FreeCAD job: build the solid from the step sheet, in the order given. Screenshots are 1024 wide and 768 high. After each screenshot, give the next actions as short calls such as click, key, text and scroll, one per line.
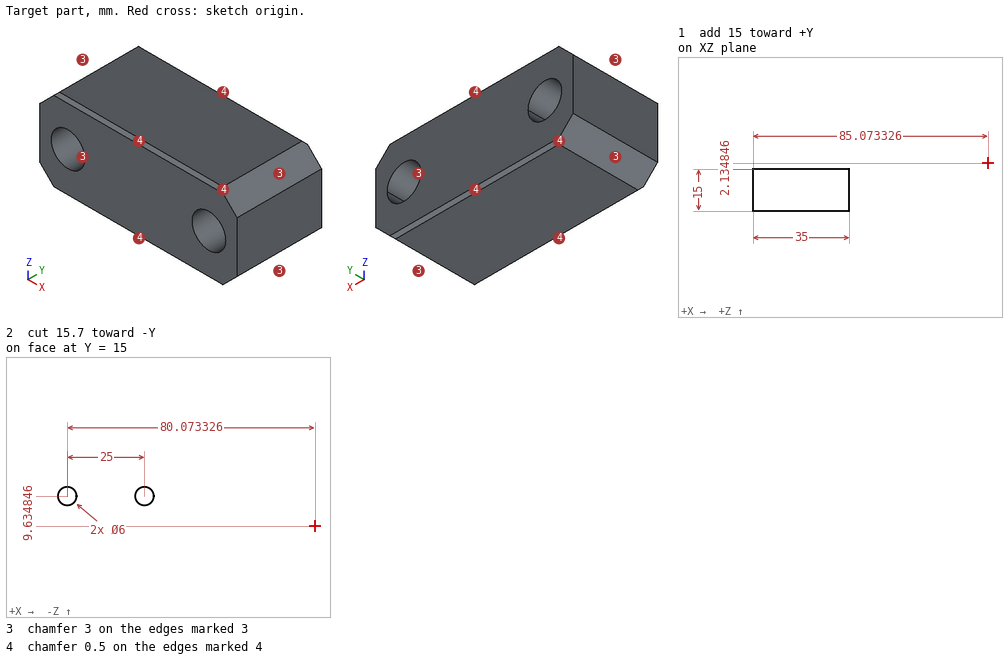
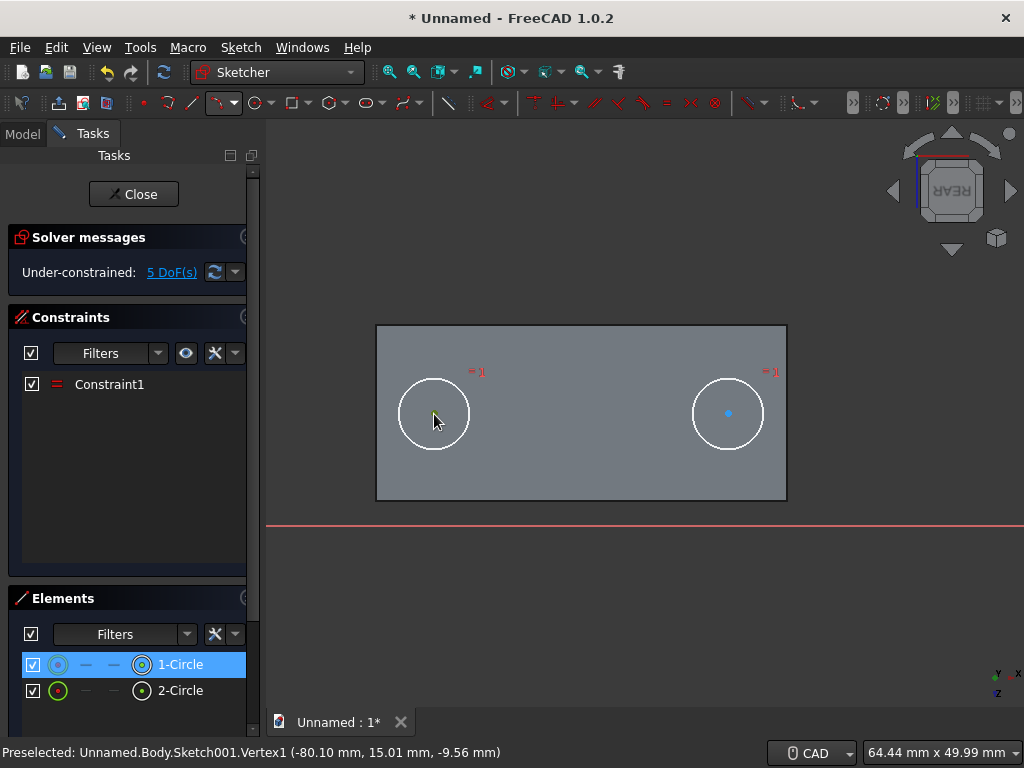
click(728, 414)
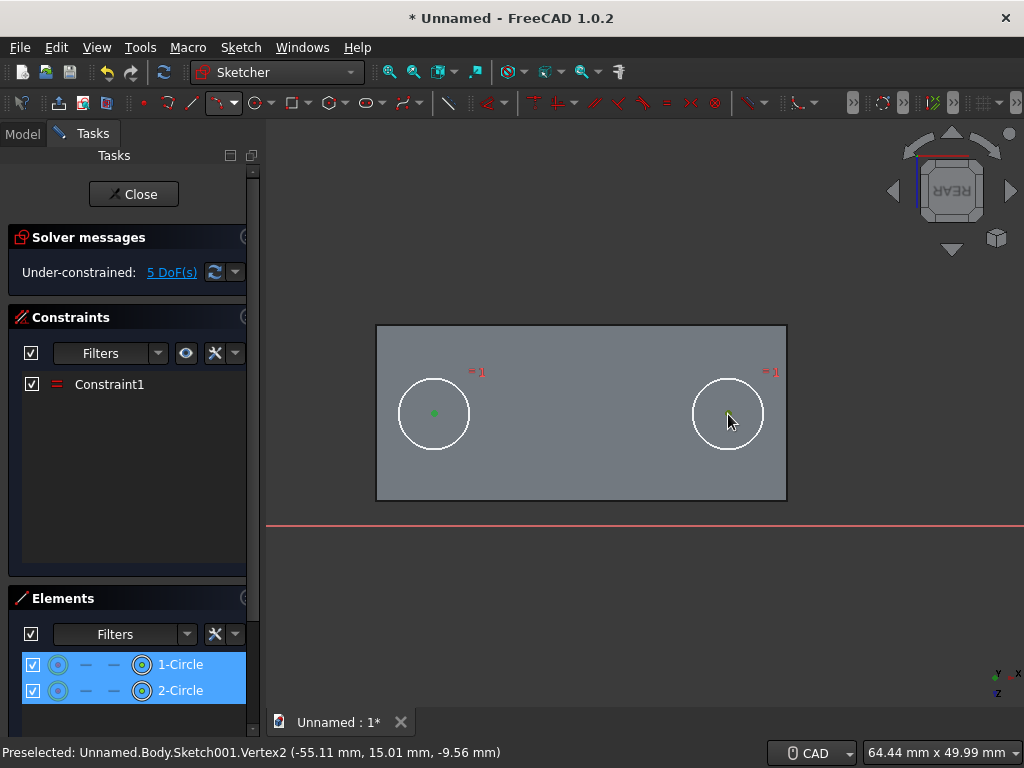
key(h)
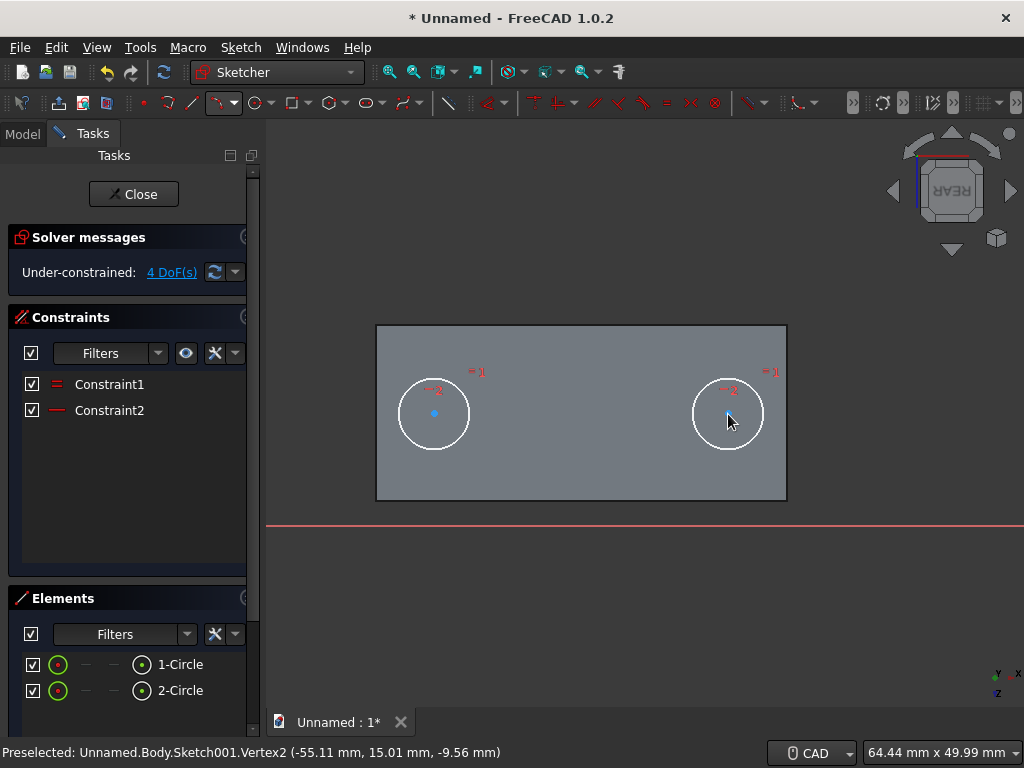
click(459, 389)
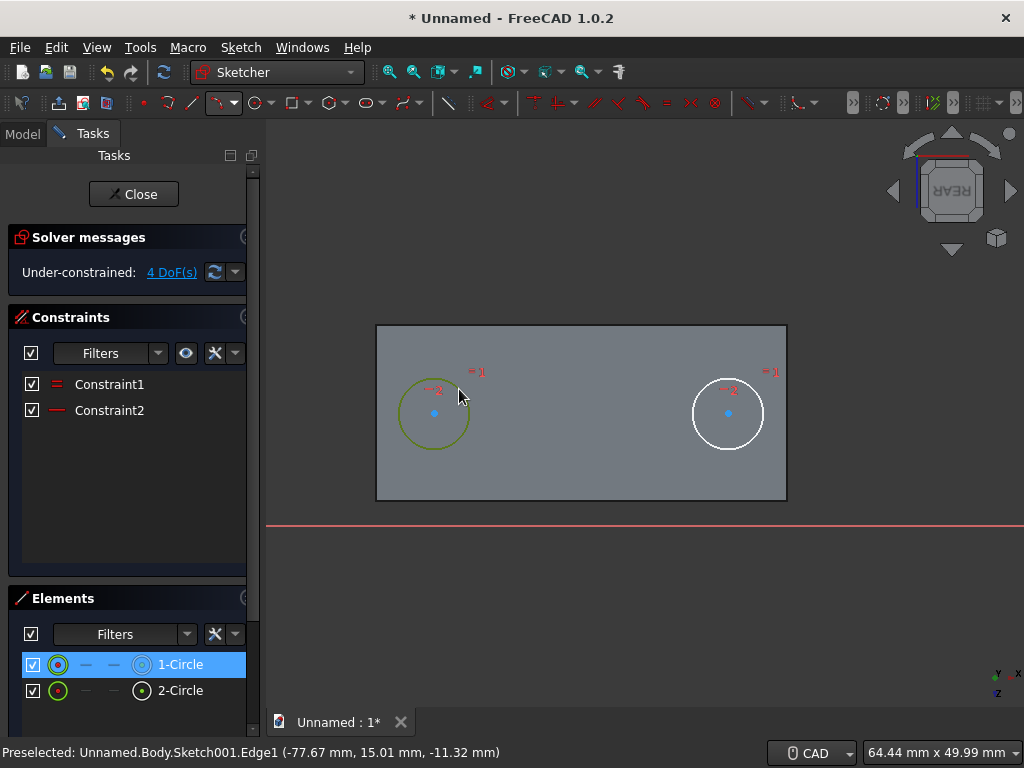
click(506, 104)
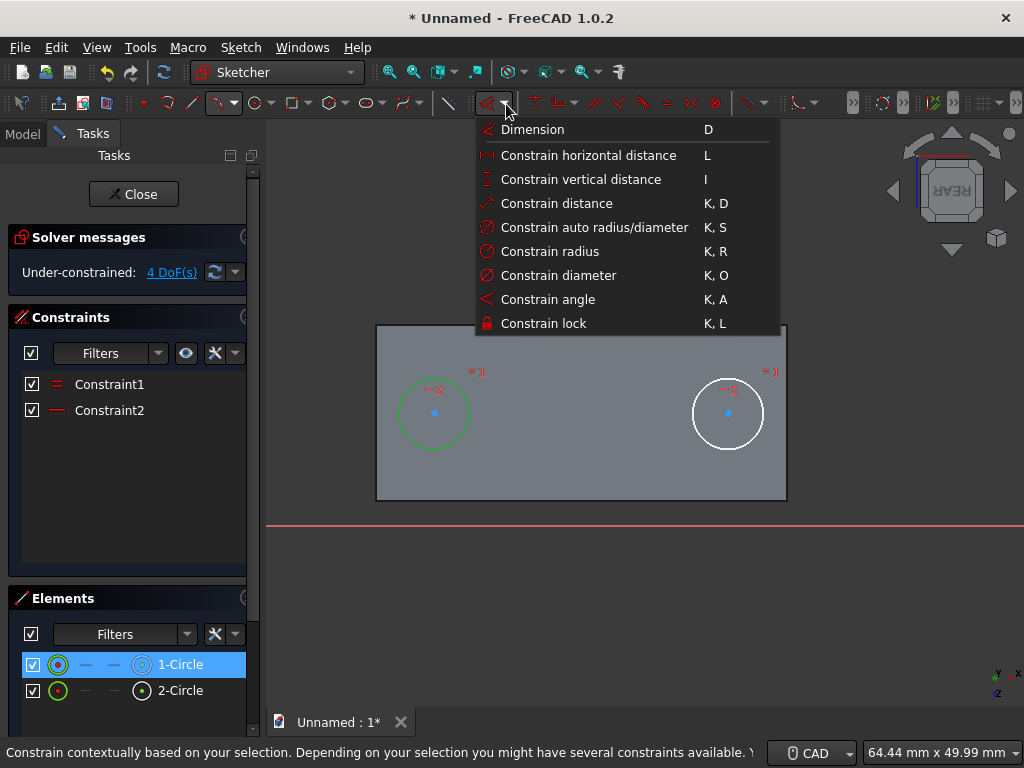
click(628, 275)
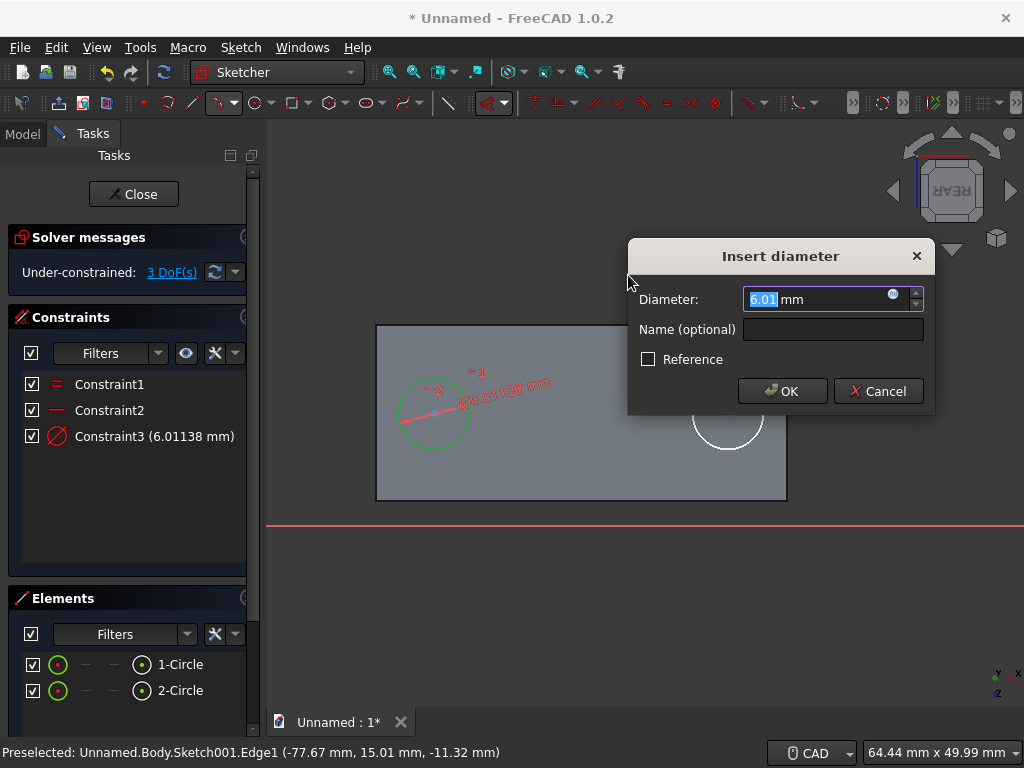
text(6)
key(Return)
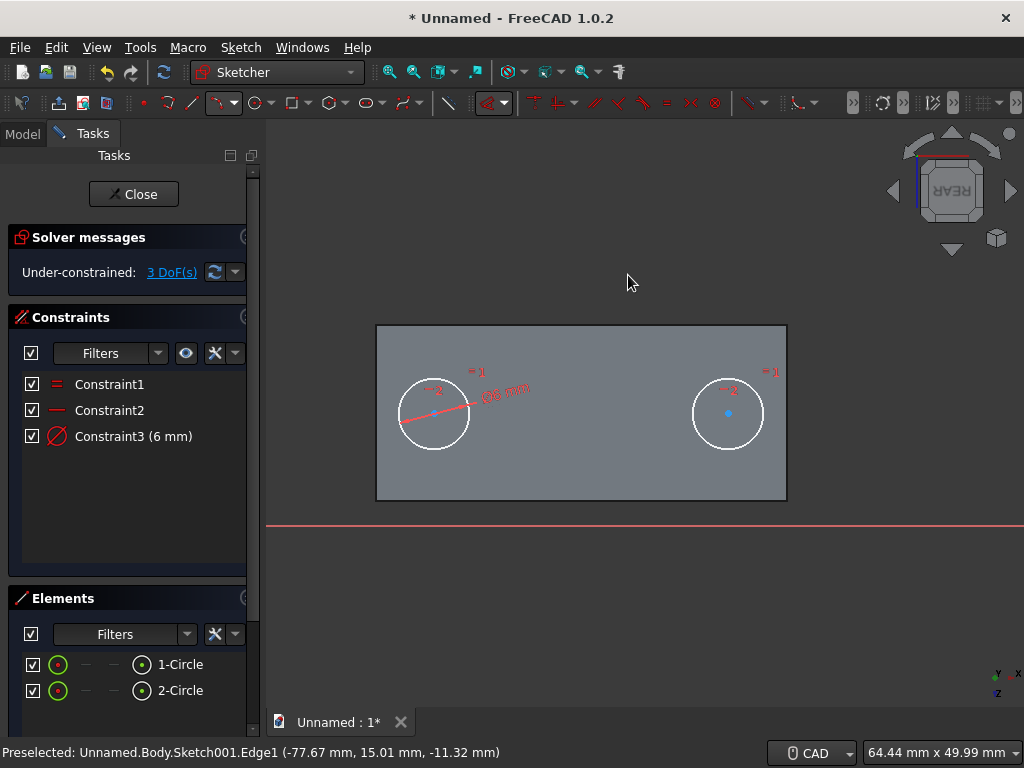
click(434, 414)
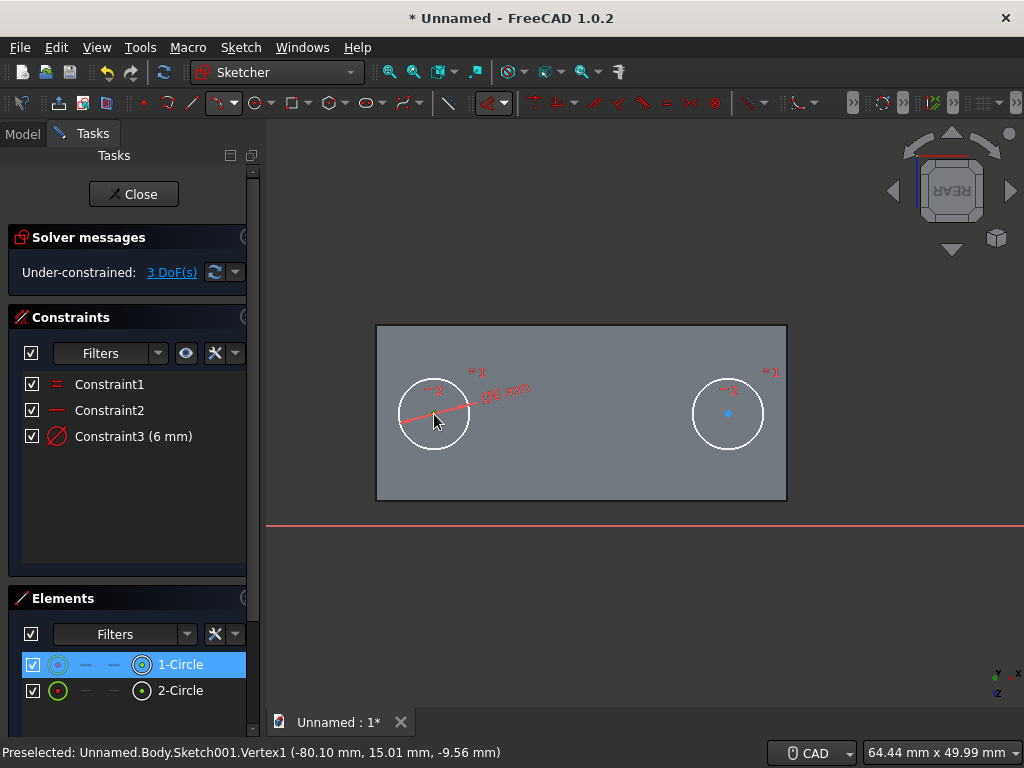
click(728, 414)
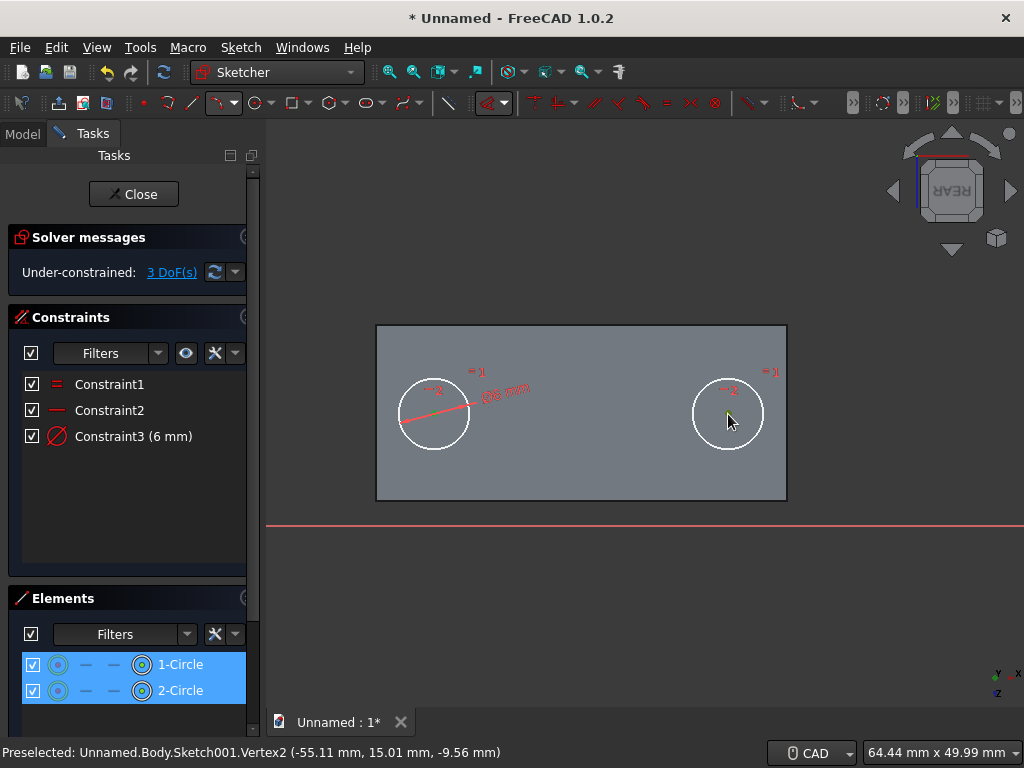
key(l)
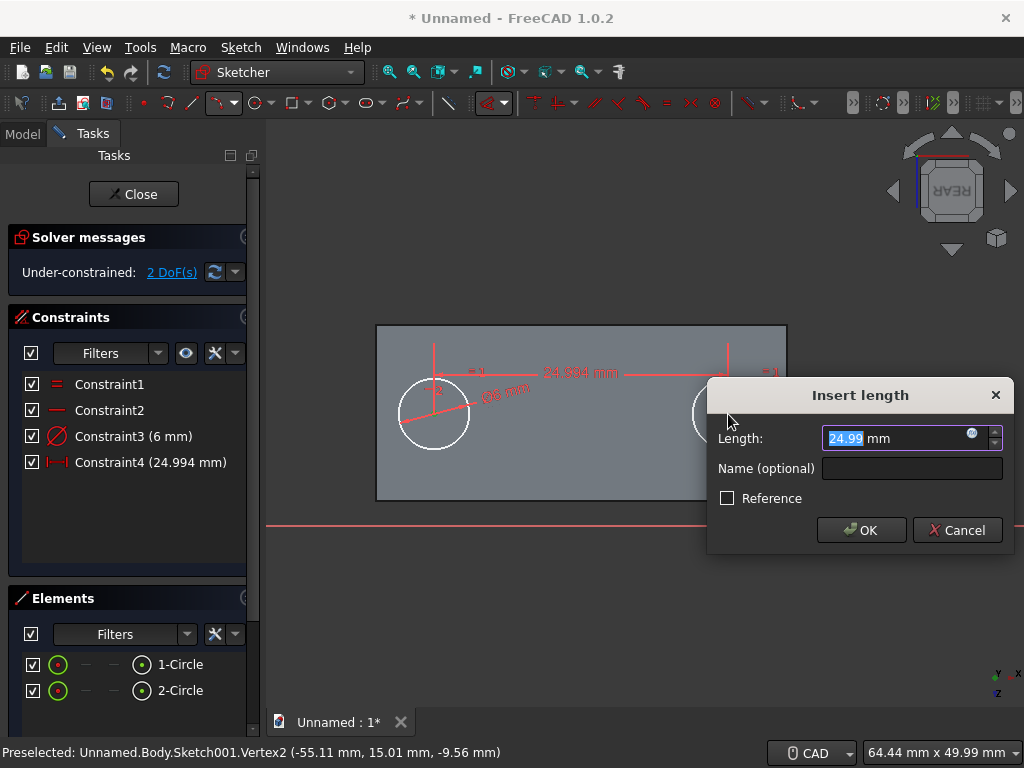
text(25)
key(Return)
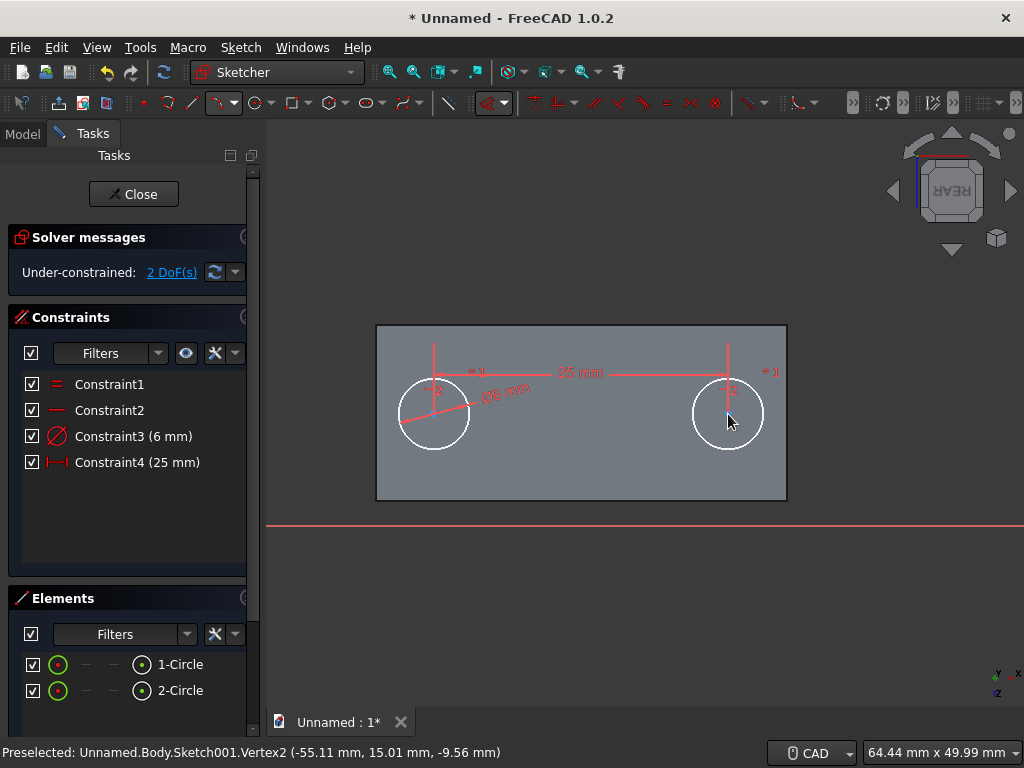
click(434, 414)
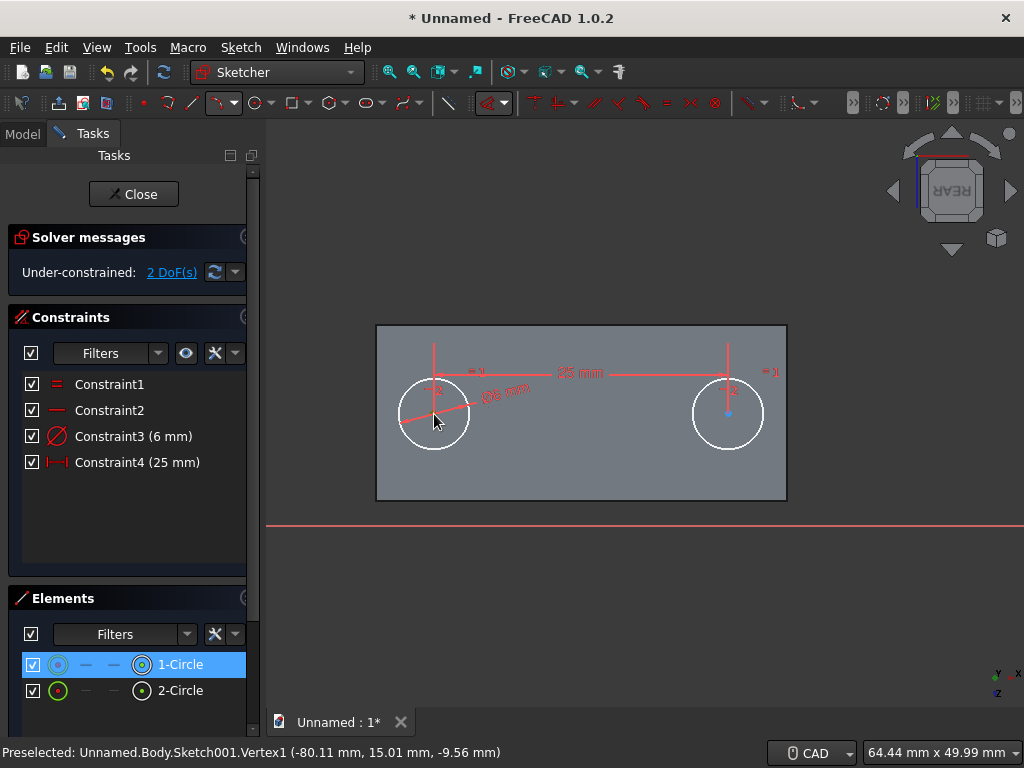
key(i)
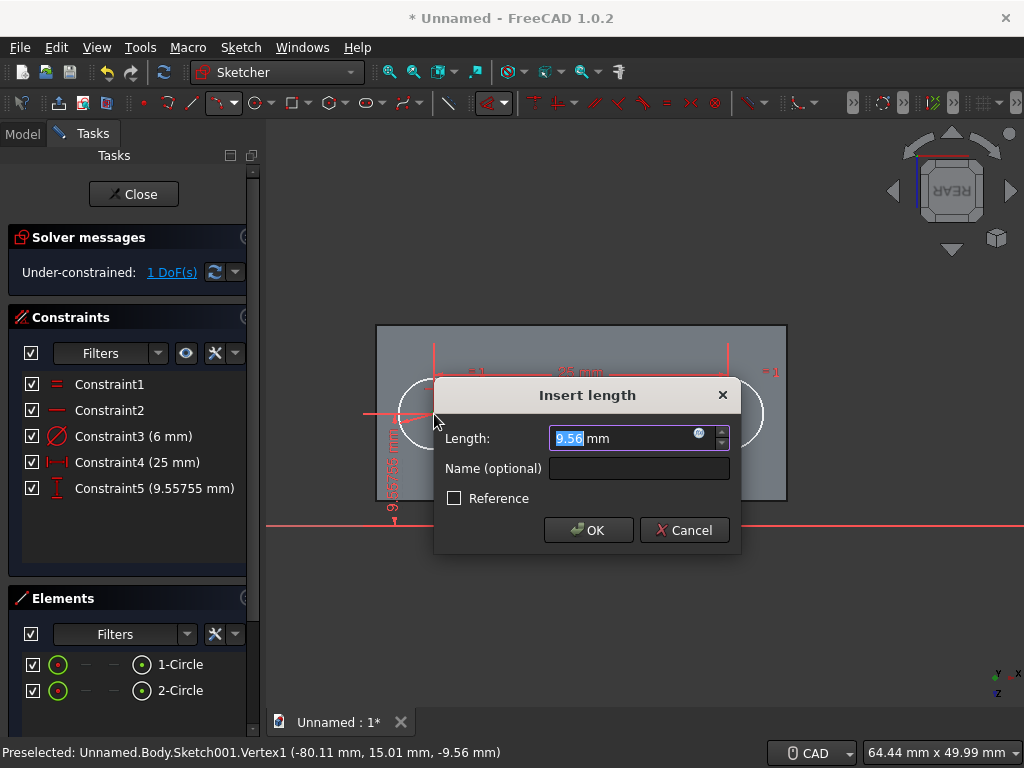
text(9.634846)
key(Return)